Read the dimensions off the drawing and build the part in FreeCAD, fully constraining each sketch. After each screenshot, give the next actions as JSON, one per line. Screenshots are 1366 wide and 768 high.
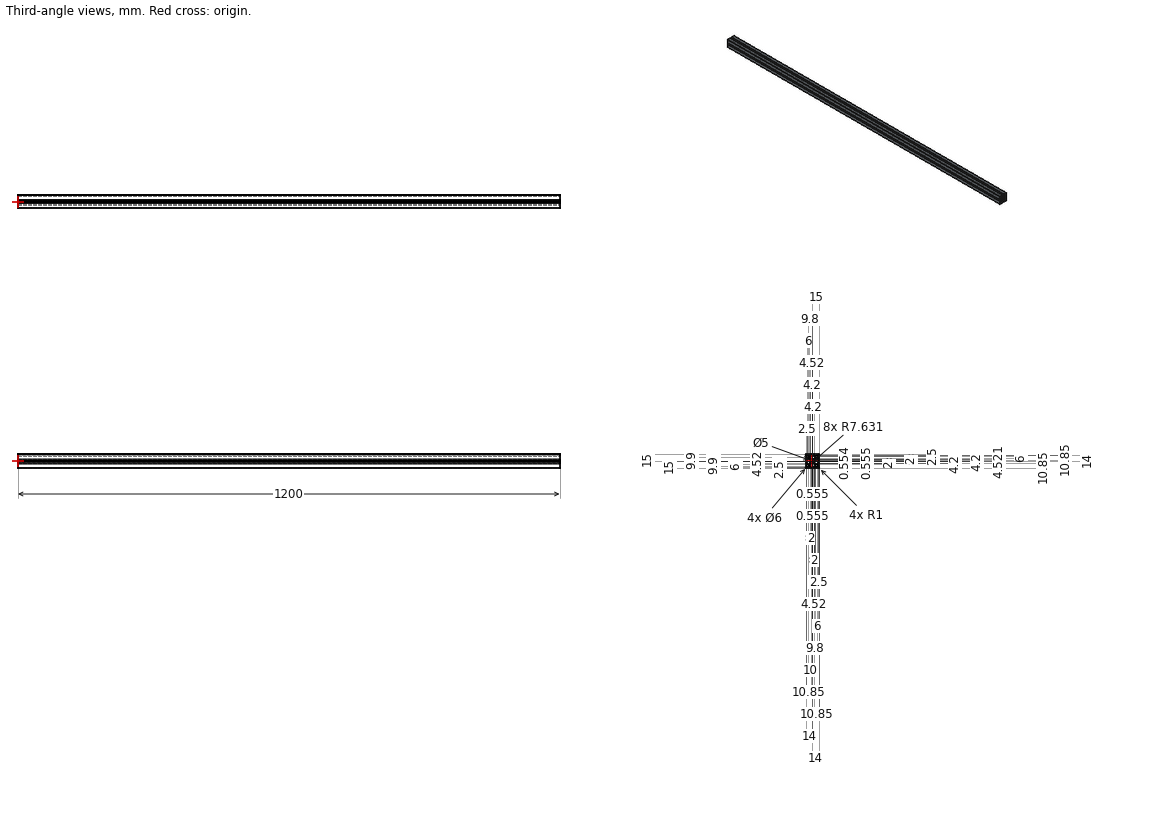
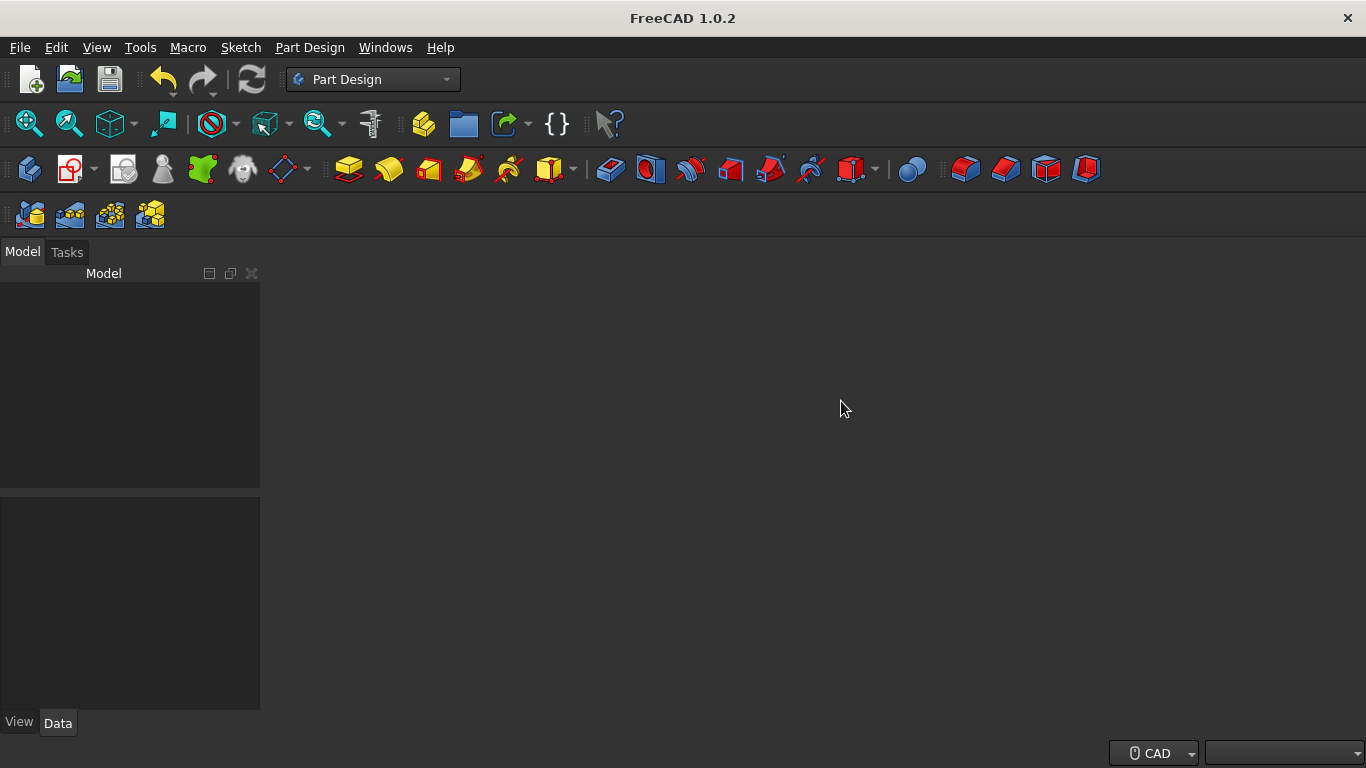
{"action": "left_click", "coordinate": [30, 80]}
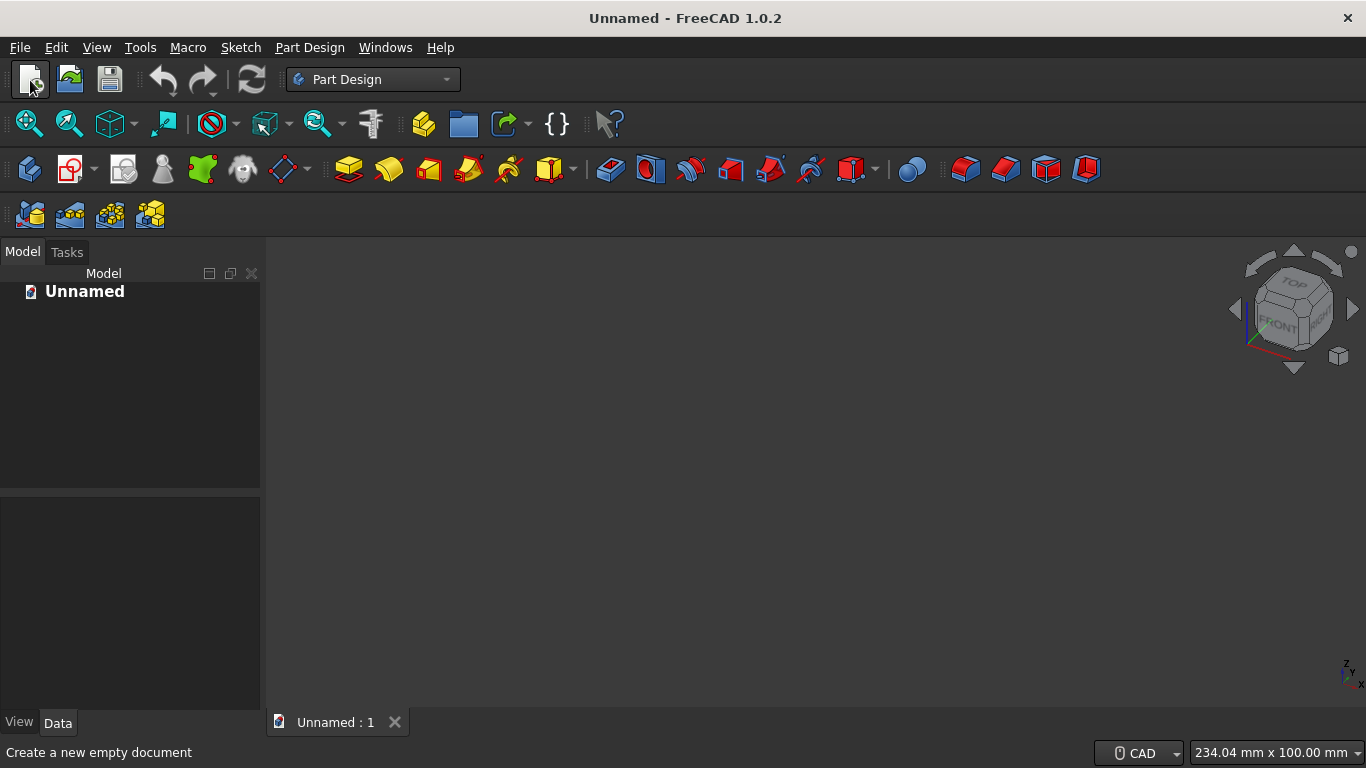
{"action": "left_click", "coordinate": [70, 170]}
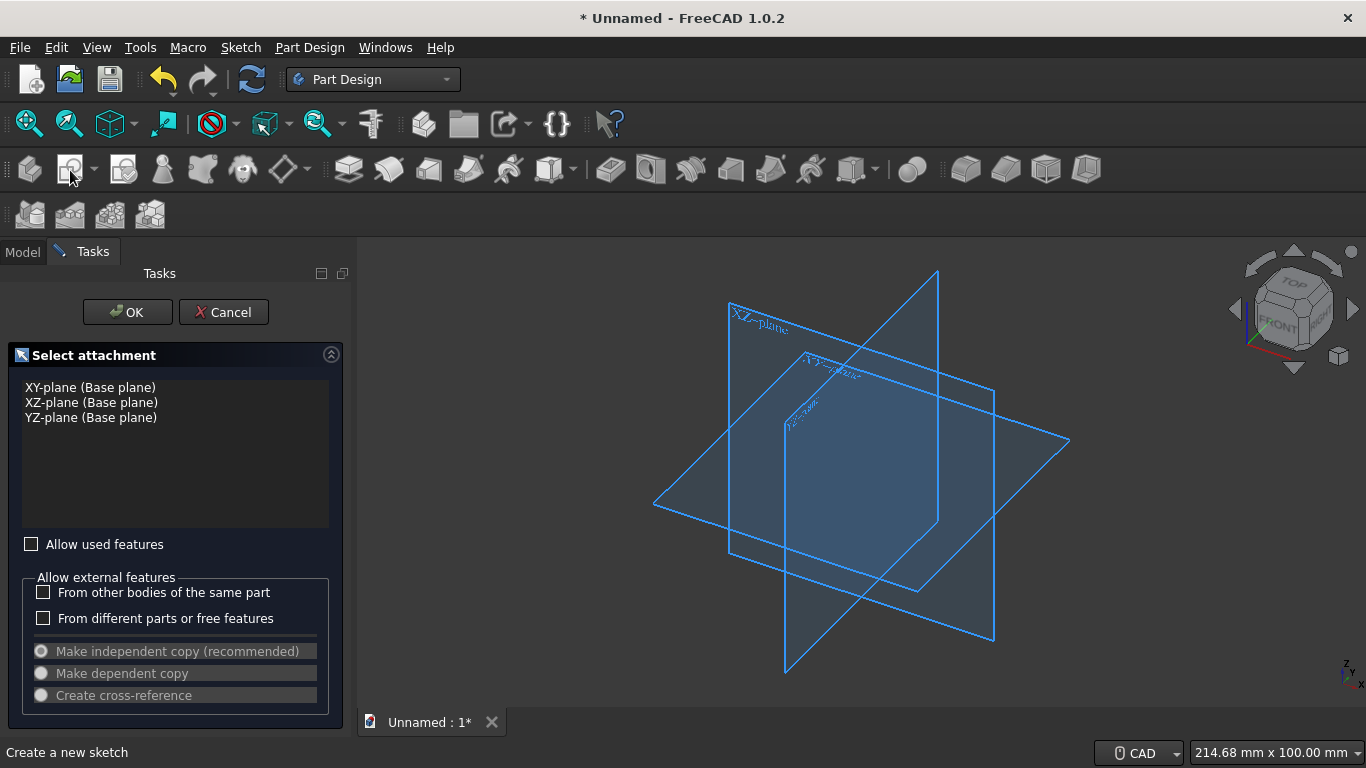
{"action": "left_click", "coordinate": [82, 418]}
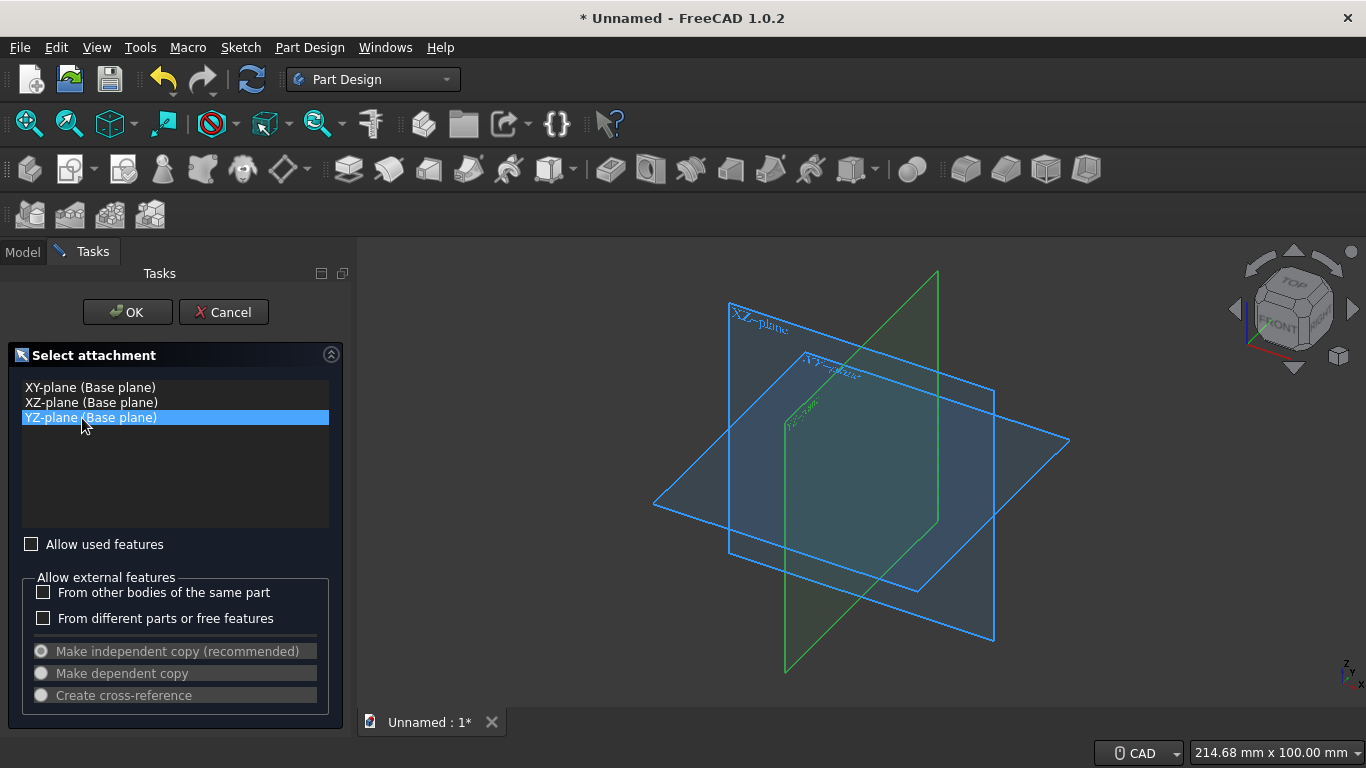
{"action": "left_click", "coordinate": [128, 312]}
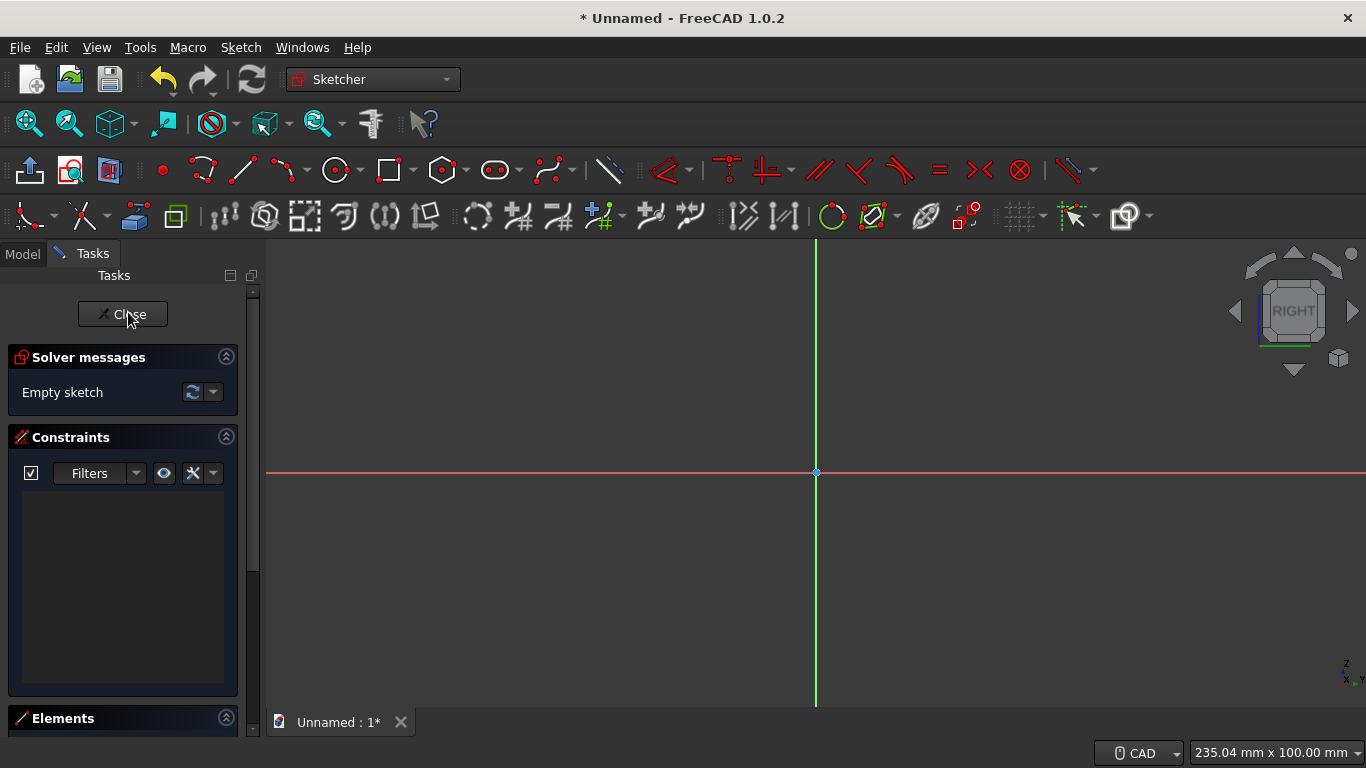
{"action": "scroll", "coordinate": [872, 473], "scroll_direction": "up", "scroll_amount": 4}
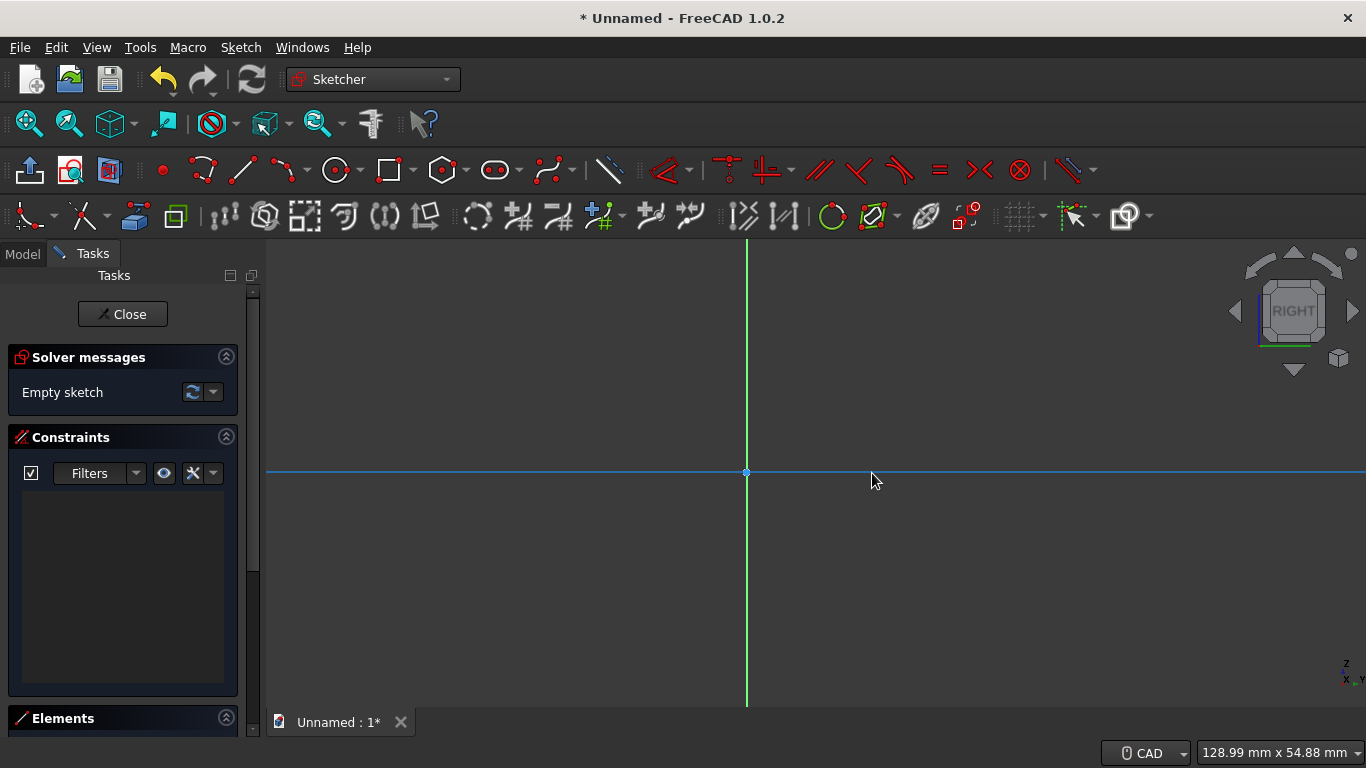
{"action": "left_click", "coordinate": [204, 170]}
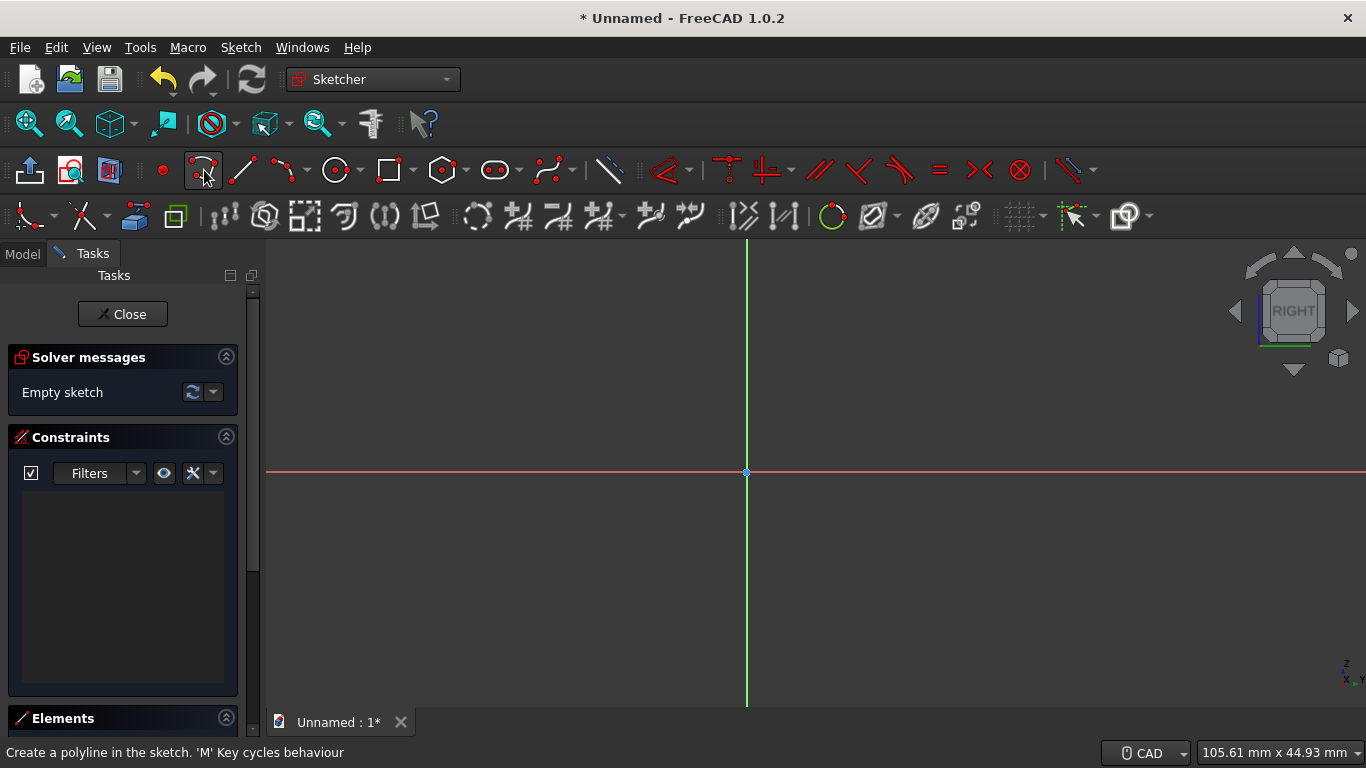
{"action": "left_click", "coordinate": [601, 629]}
{"action": "left_click", "coordinate": [714, 629]}
{"action": "left_click", "coordinate": [714, 603]}
{"action": "left_click", "coordinate": [693, 603]}
{"action": "left_click", "coordinate": [693, 540]}
{"action": "right_click", "coordinate": [693, 540]}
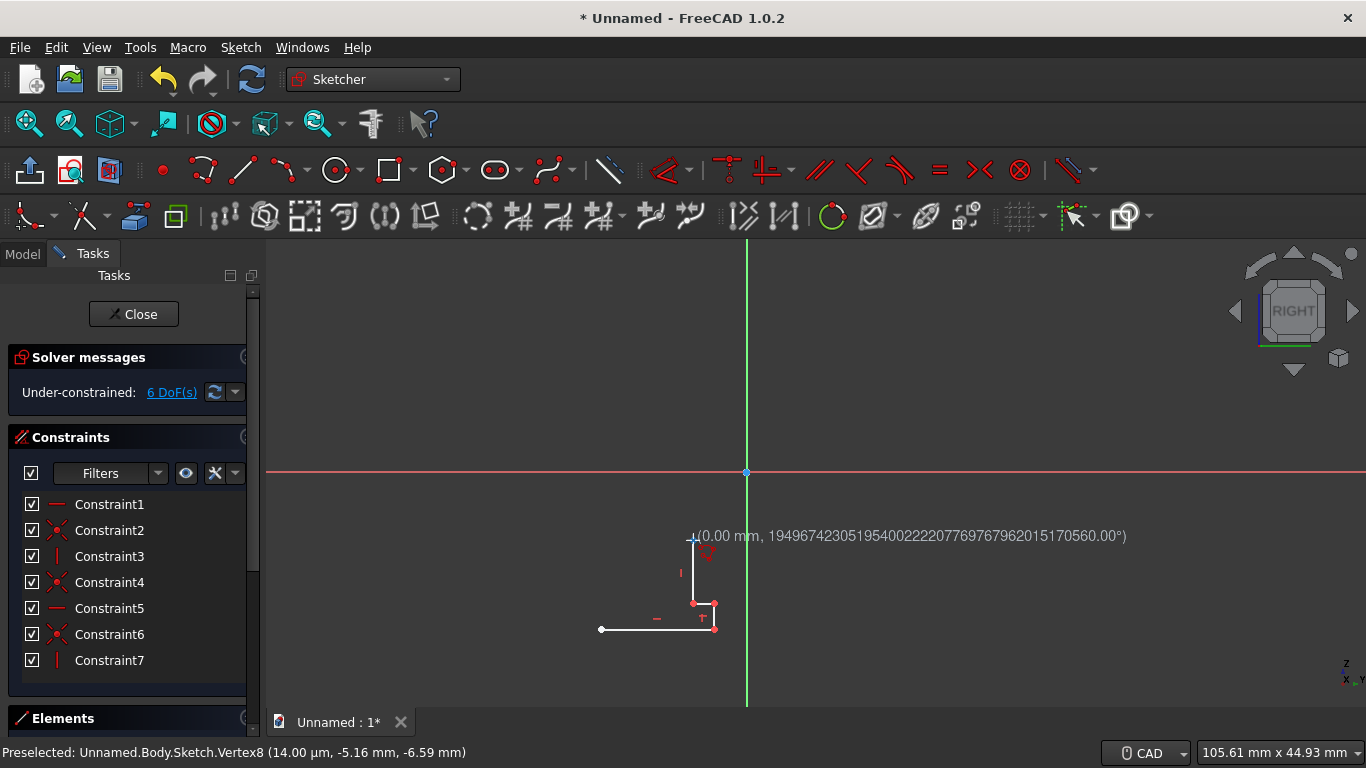
{"action": "scroll", "coordinate": [741, 519], "scroll_direction": "up", "scroll_amount": 6}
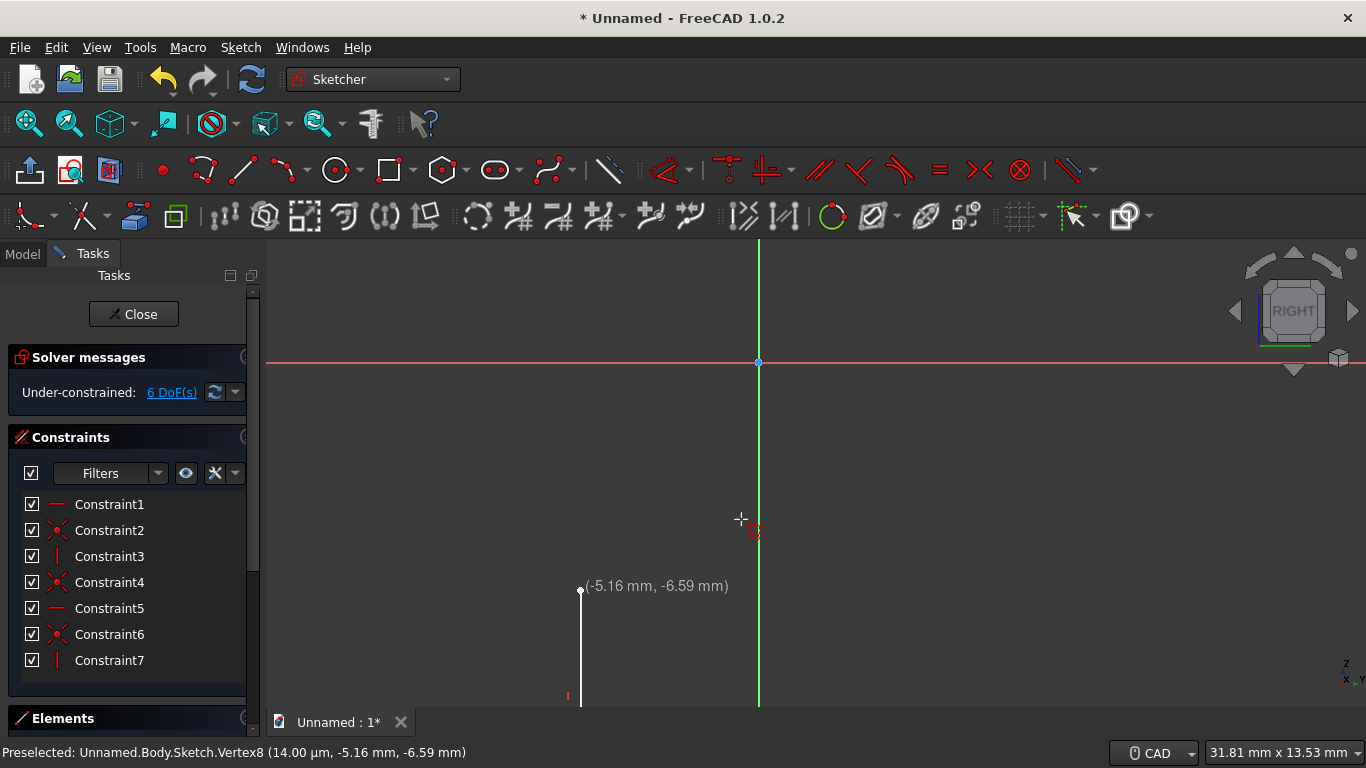
{"action": "left_click", "coordinate": [740, 519]}
{"action": "left_click", "coordinate": [759, 508]}
{"action": "left_click", "coordinate": [778, 519]}
{"action": "right_click", "coordinate": [778, 519]}